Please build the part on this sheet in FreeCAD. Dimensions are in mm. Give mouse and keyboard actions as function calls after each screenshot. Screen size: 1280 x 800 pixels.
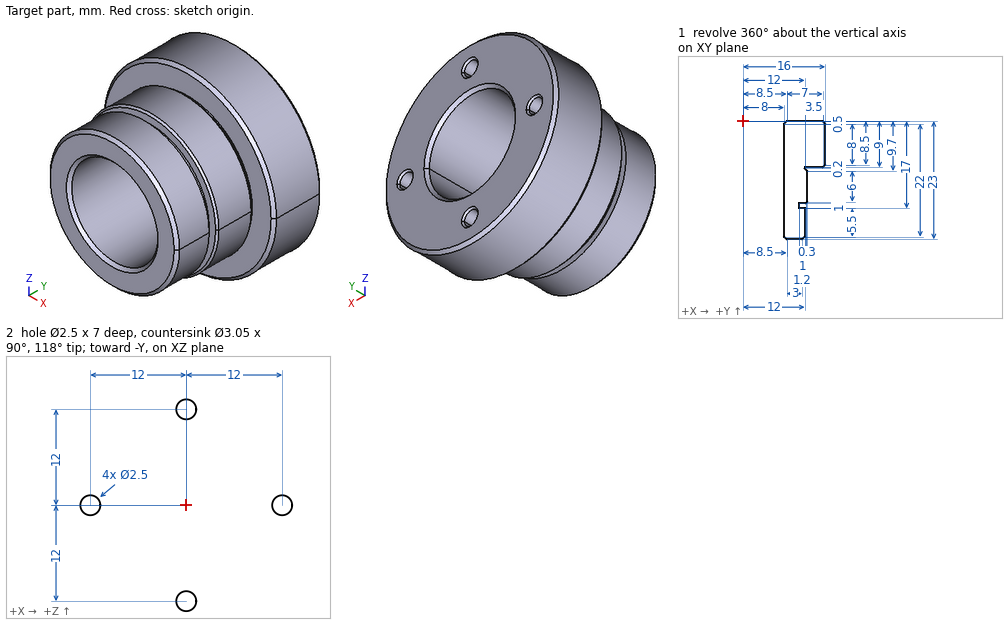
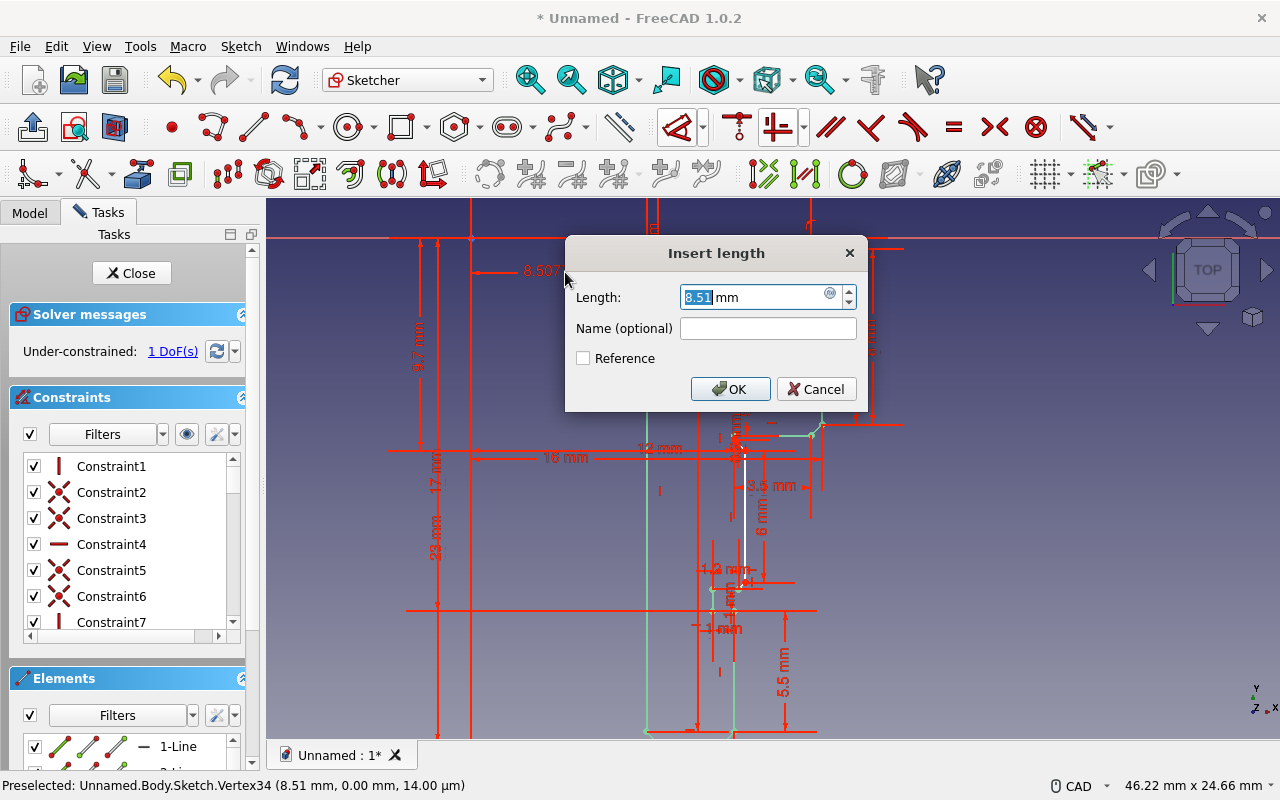
text(8.5)
key(Return)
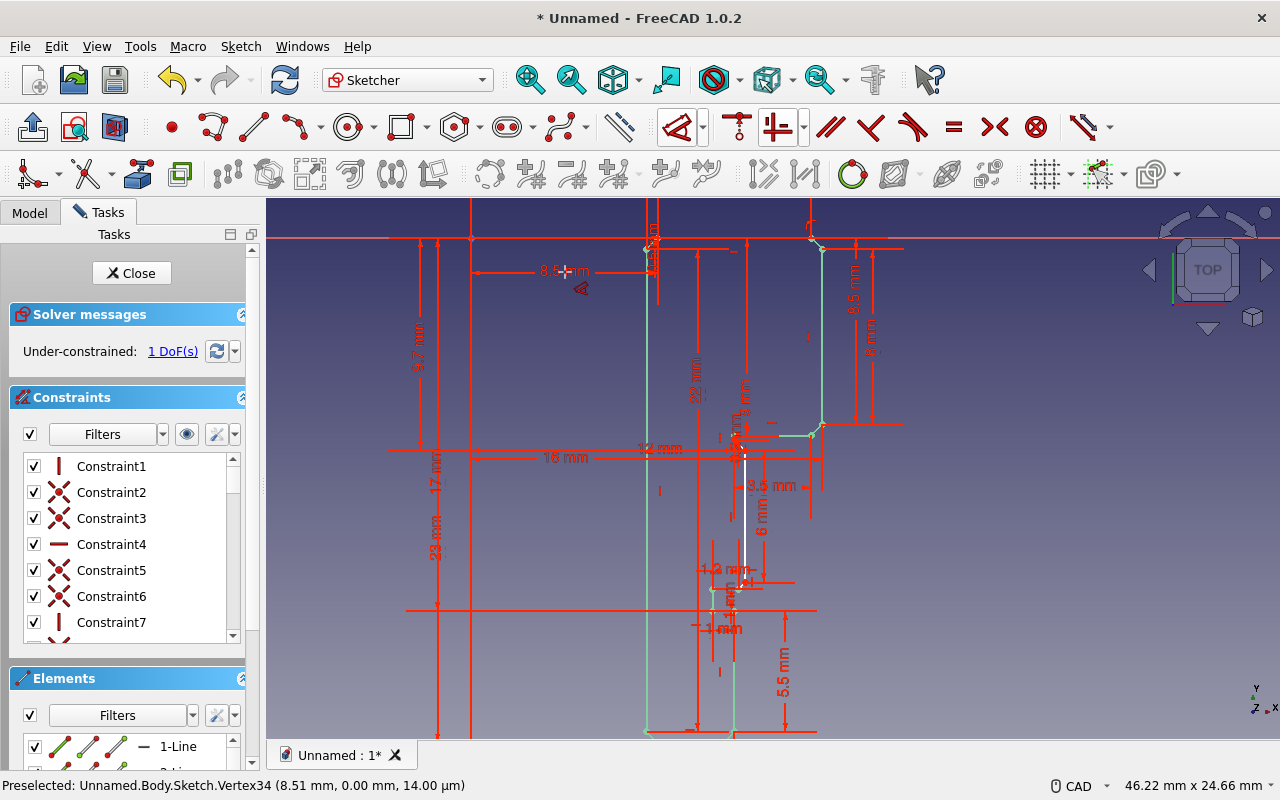
scroll(742, 586, up, 9)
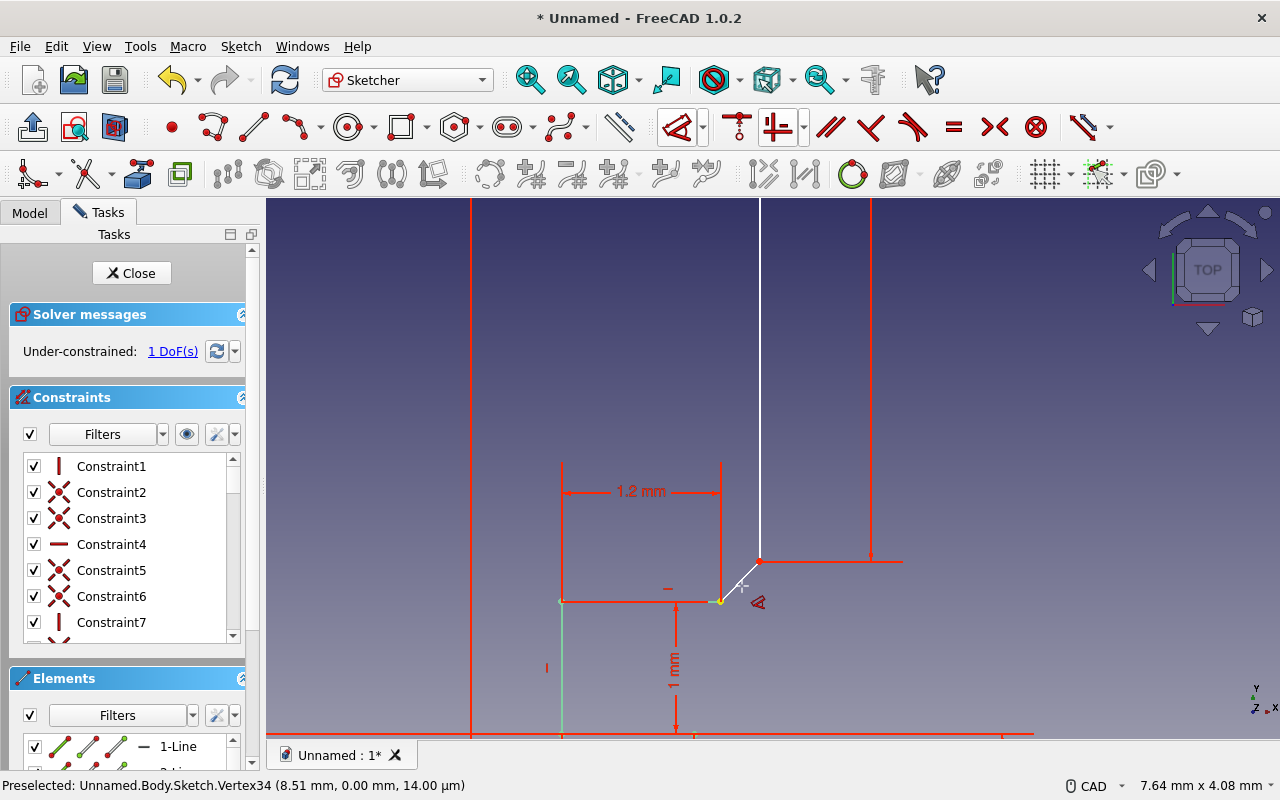
click(740, 582)
click(740, 636)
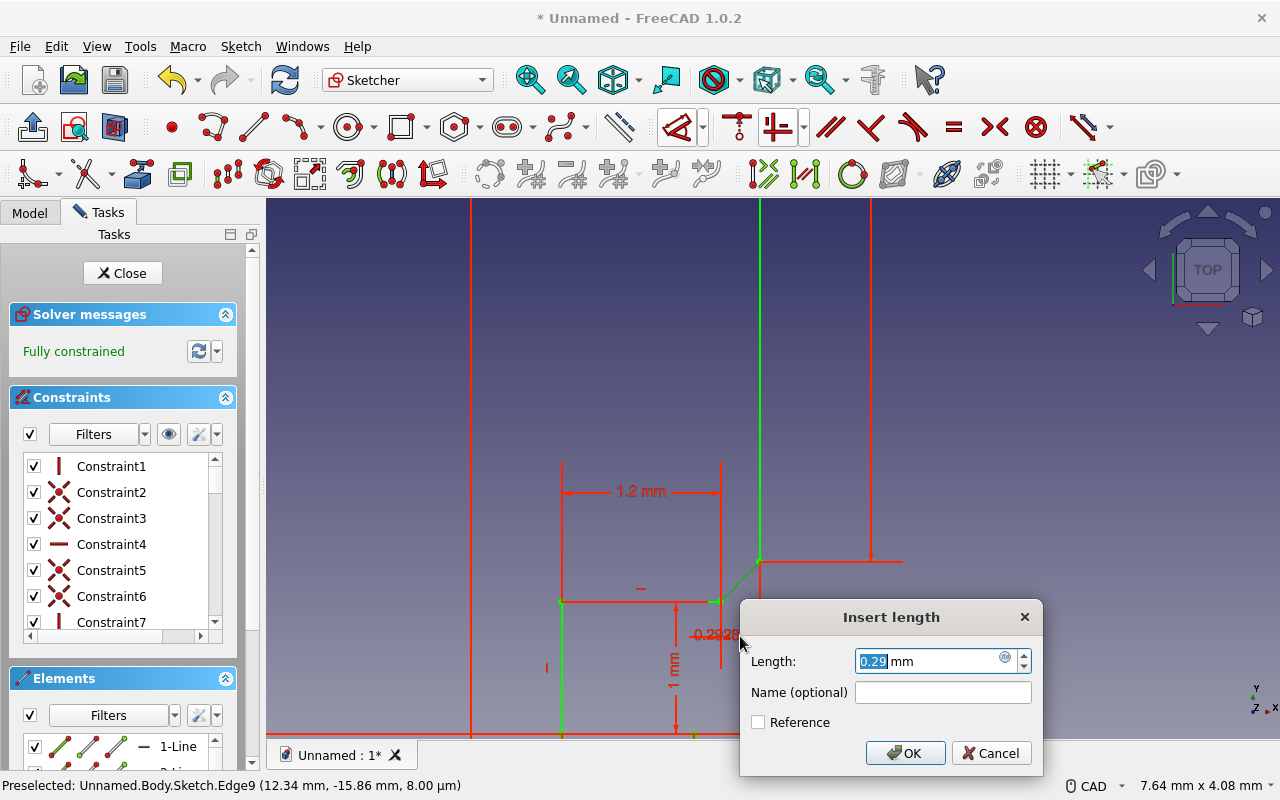
text(0.3)
key(Return)
key(Escape)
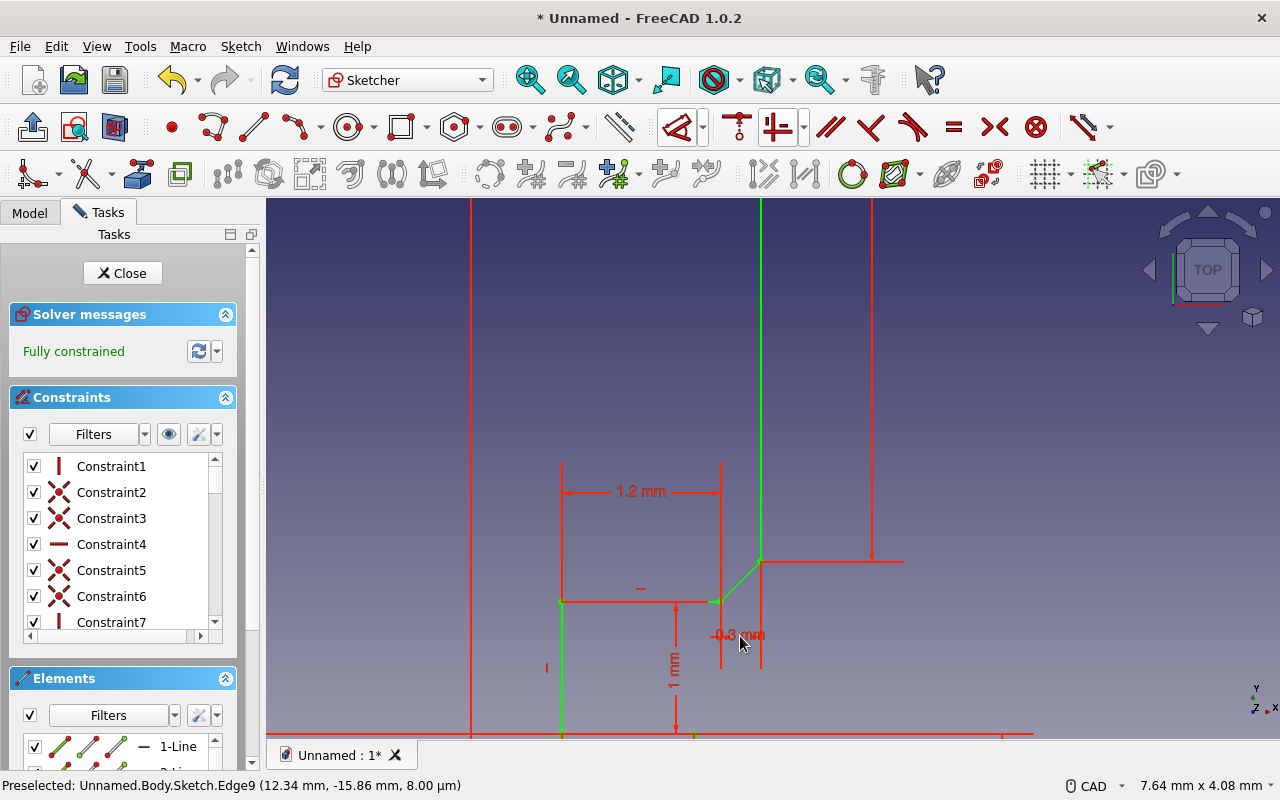
click(123, 273)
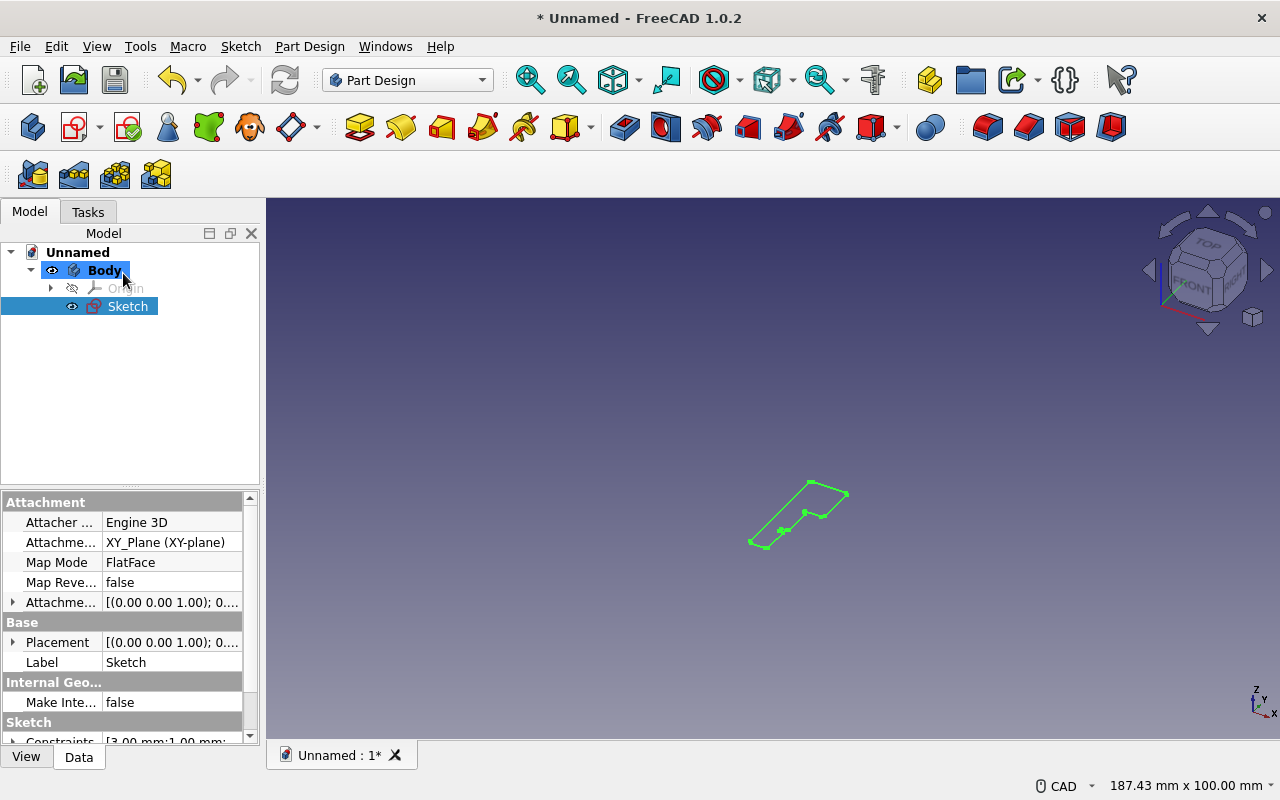
click(401, 128)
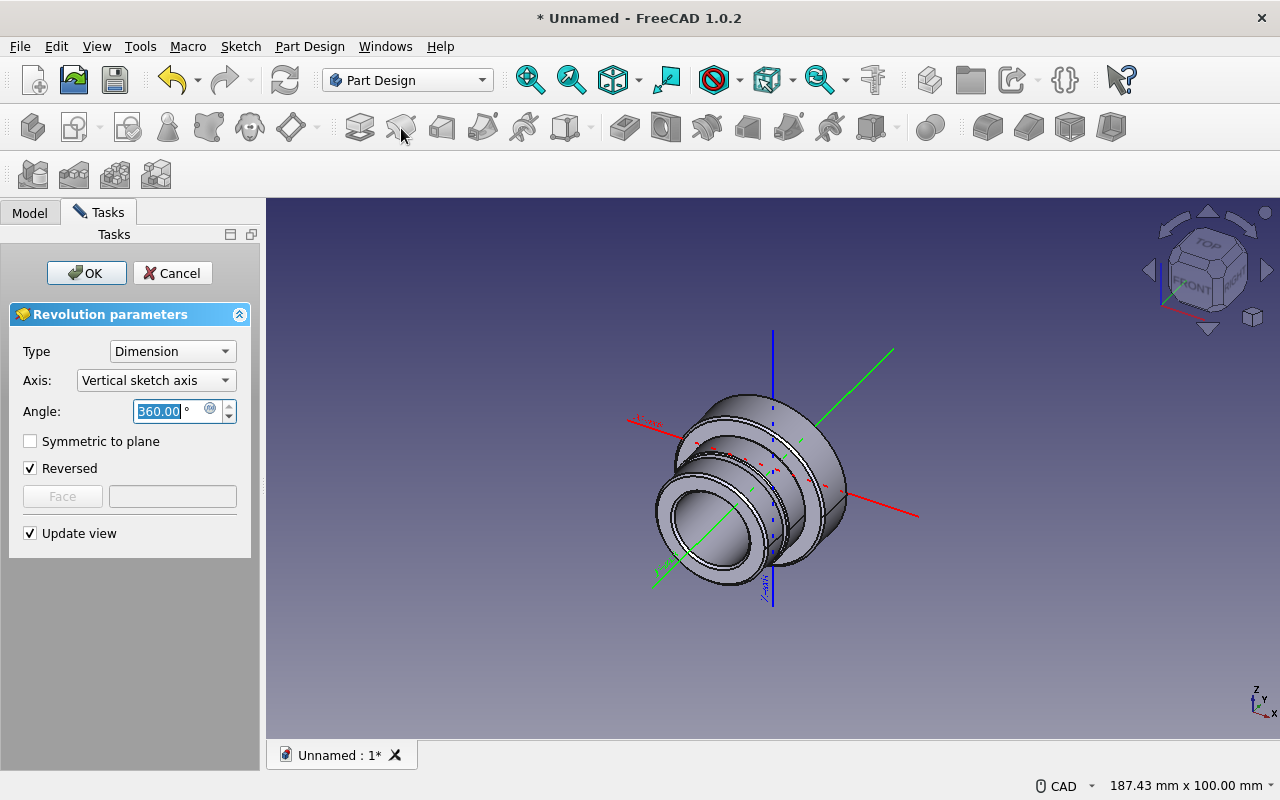
click(87, 273)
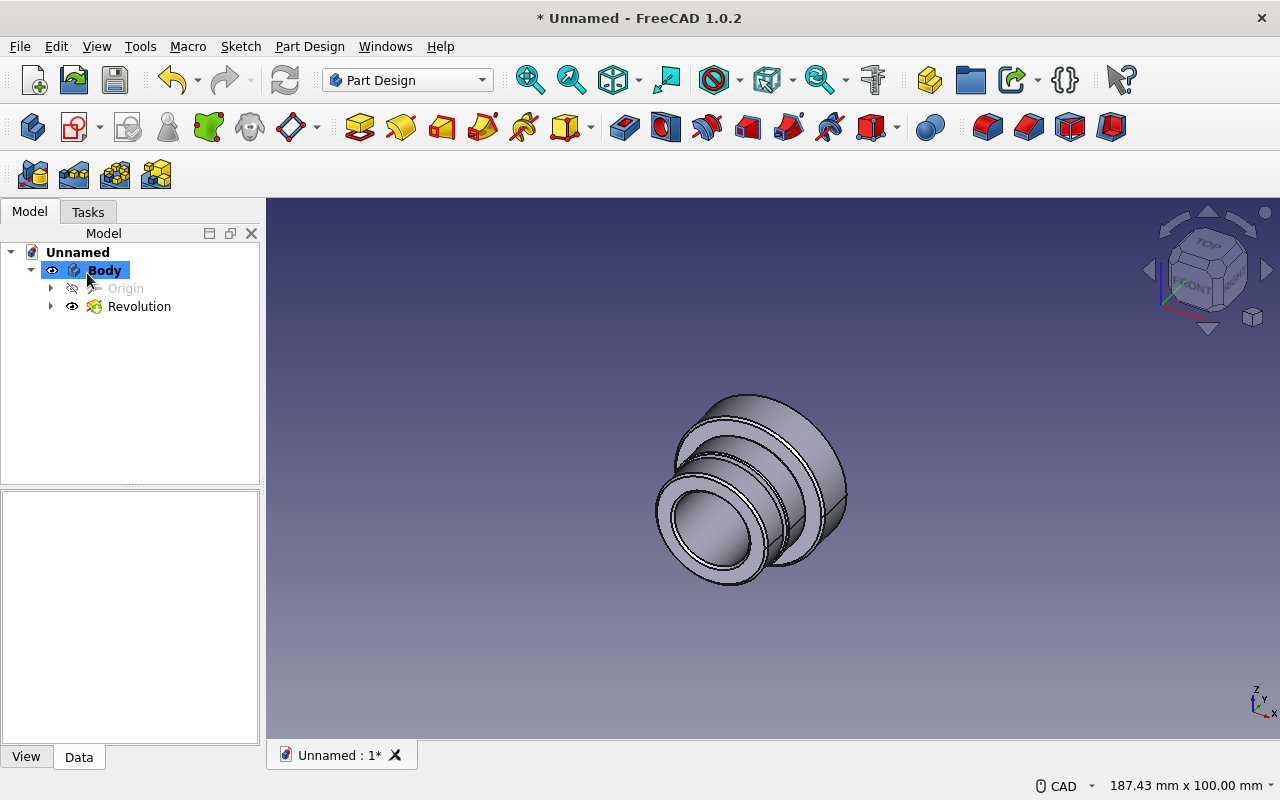
click(74, 128)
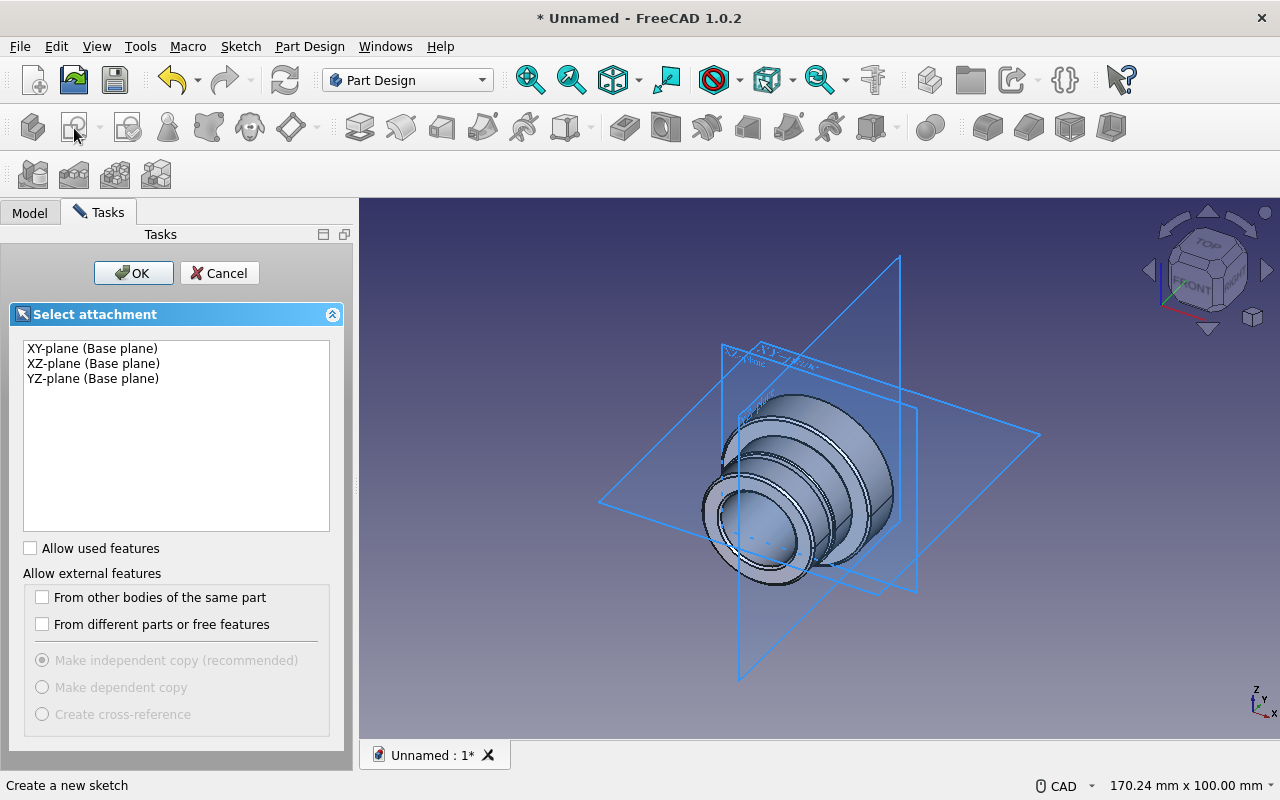
click(84, 364)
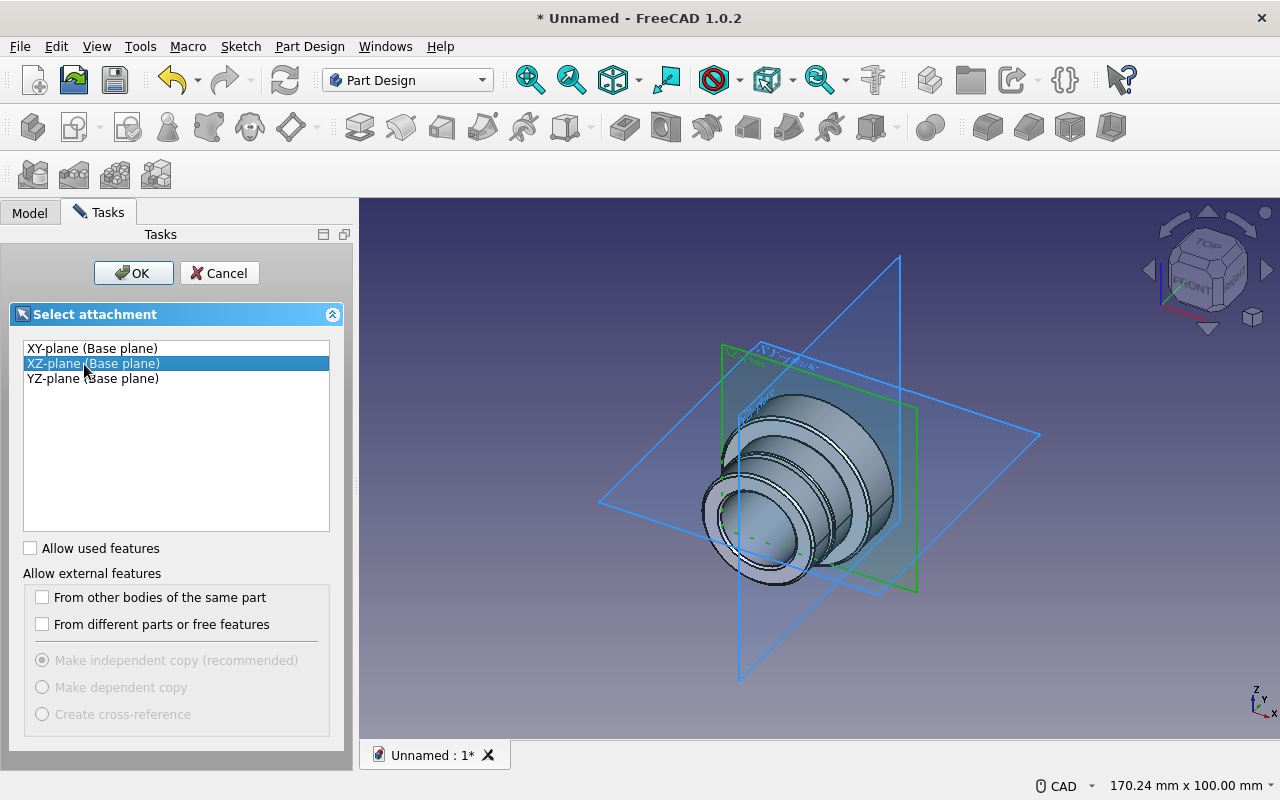
click(134, 273)